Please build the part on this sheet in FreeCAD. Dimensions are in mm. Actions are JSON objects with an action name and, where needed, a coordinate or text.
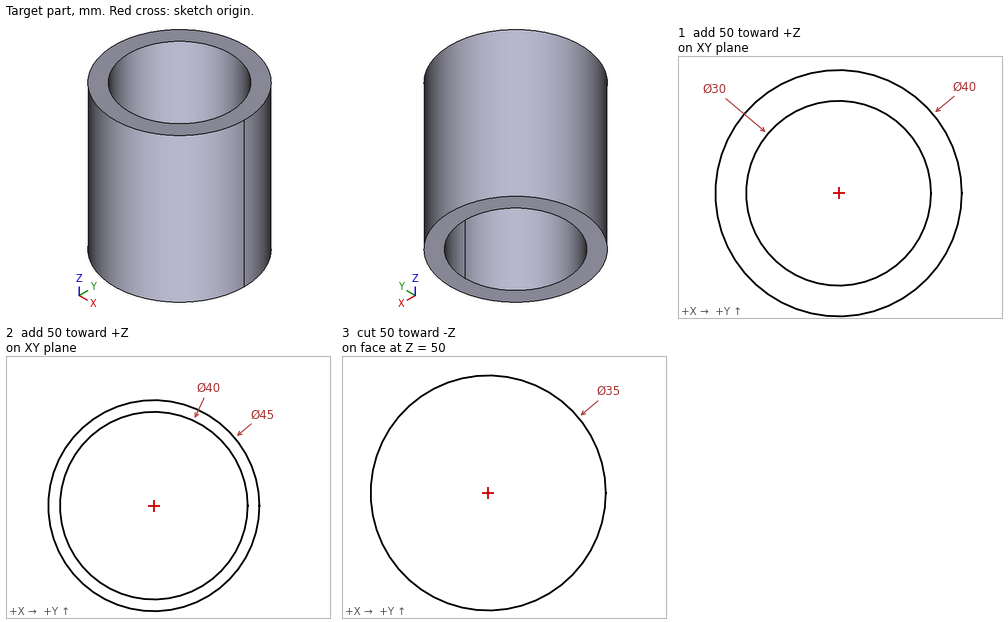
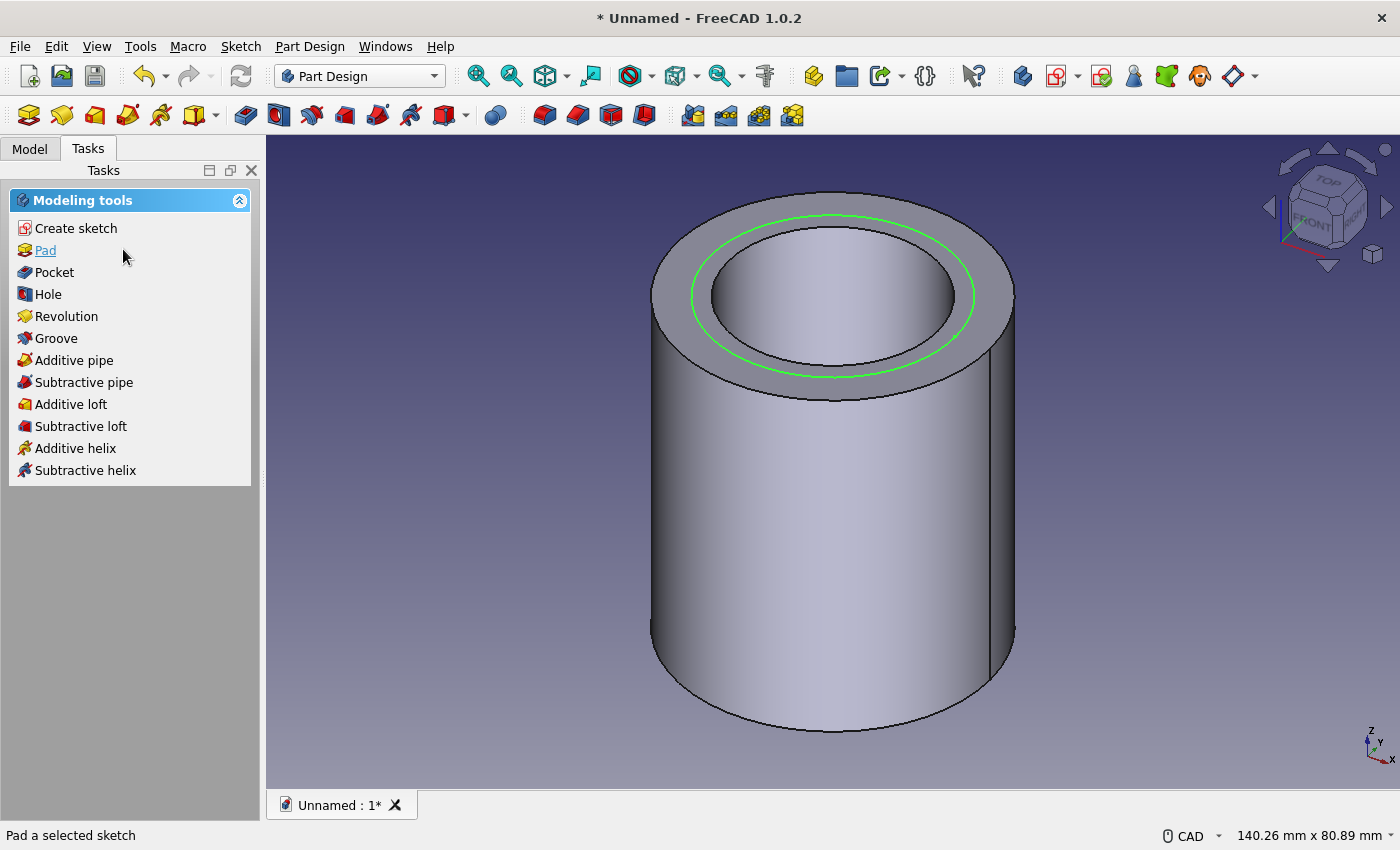
{"action": "left_click", "coordinate": [246, 116]}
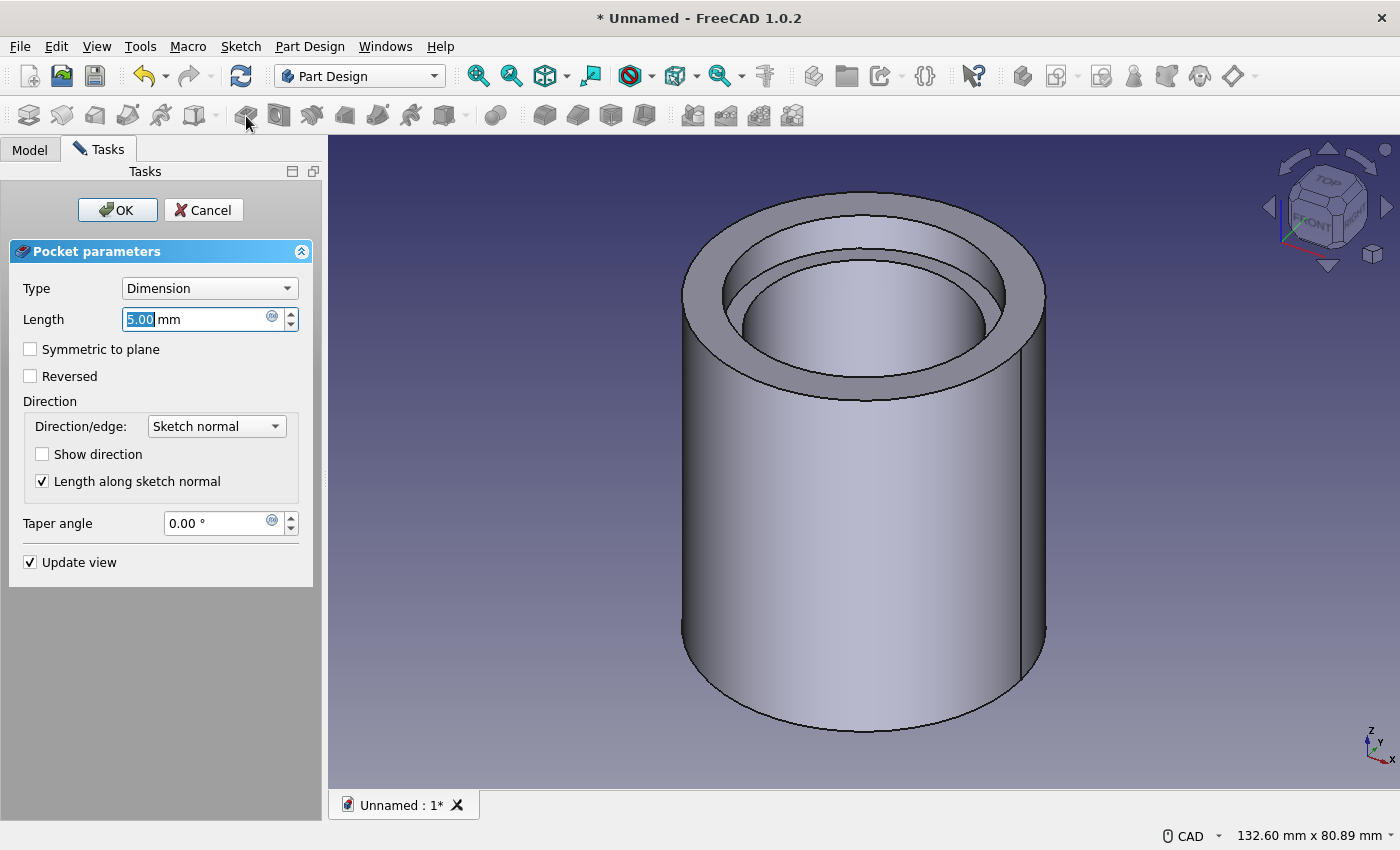
{"action": "type", "text": "50"}
{"action": "key", "text": "Tab"}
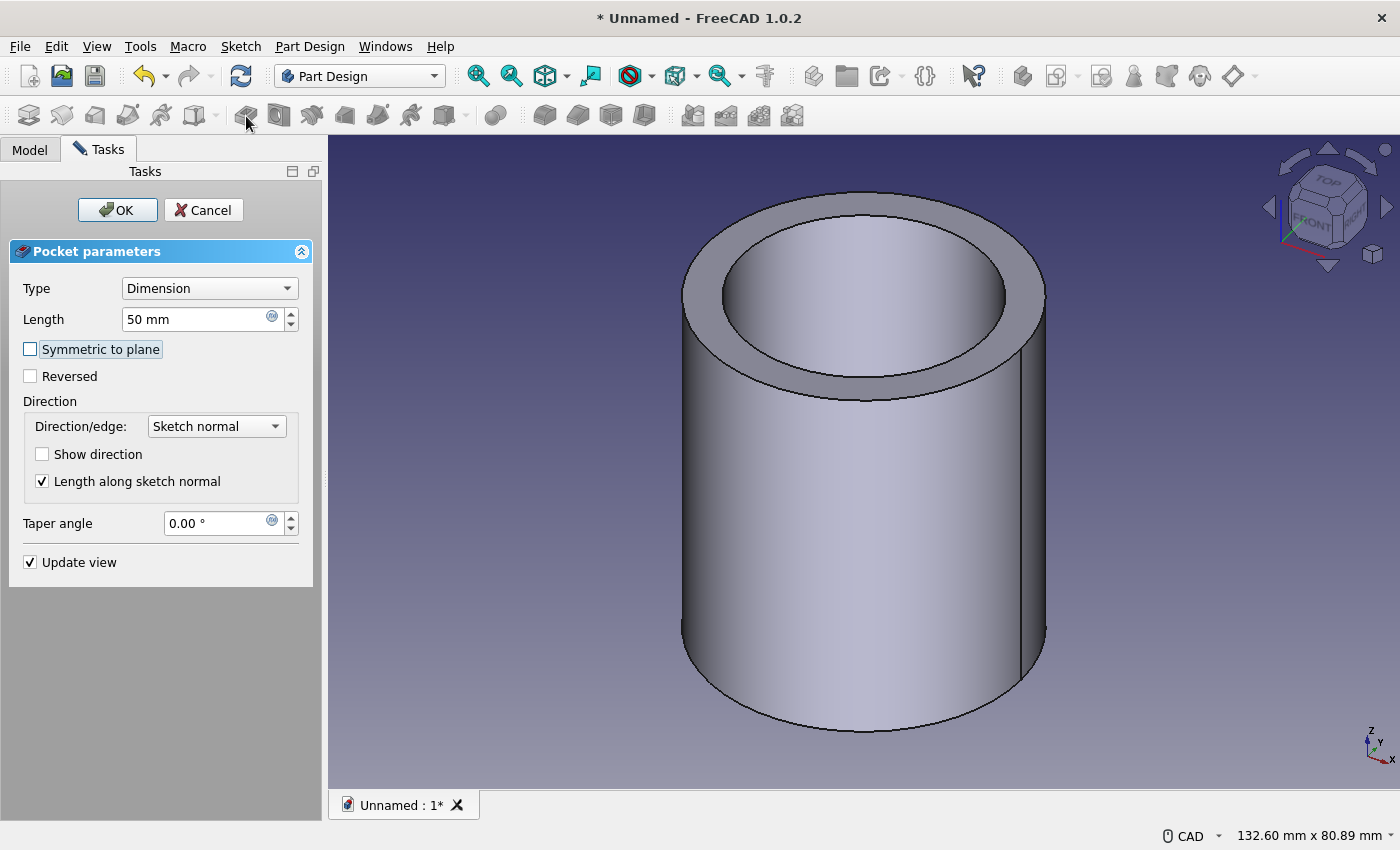
{"action": "left_click", "coordinate": [118, 210]}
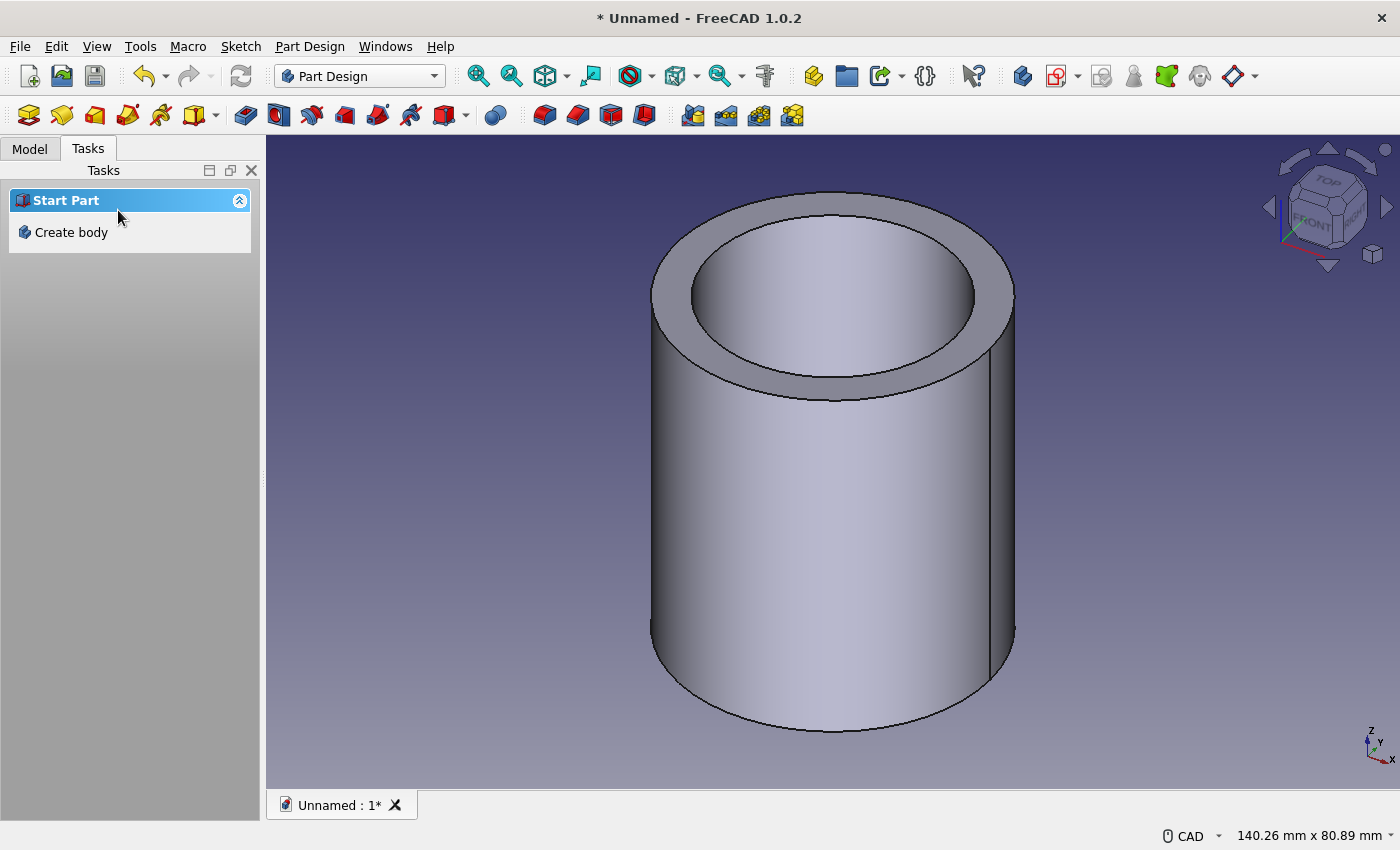
{"action": "key", "text": "0"}